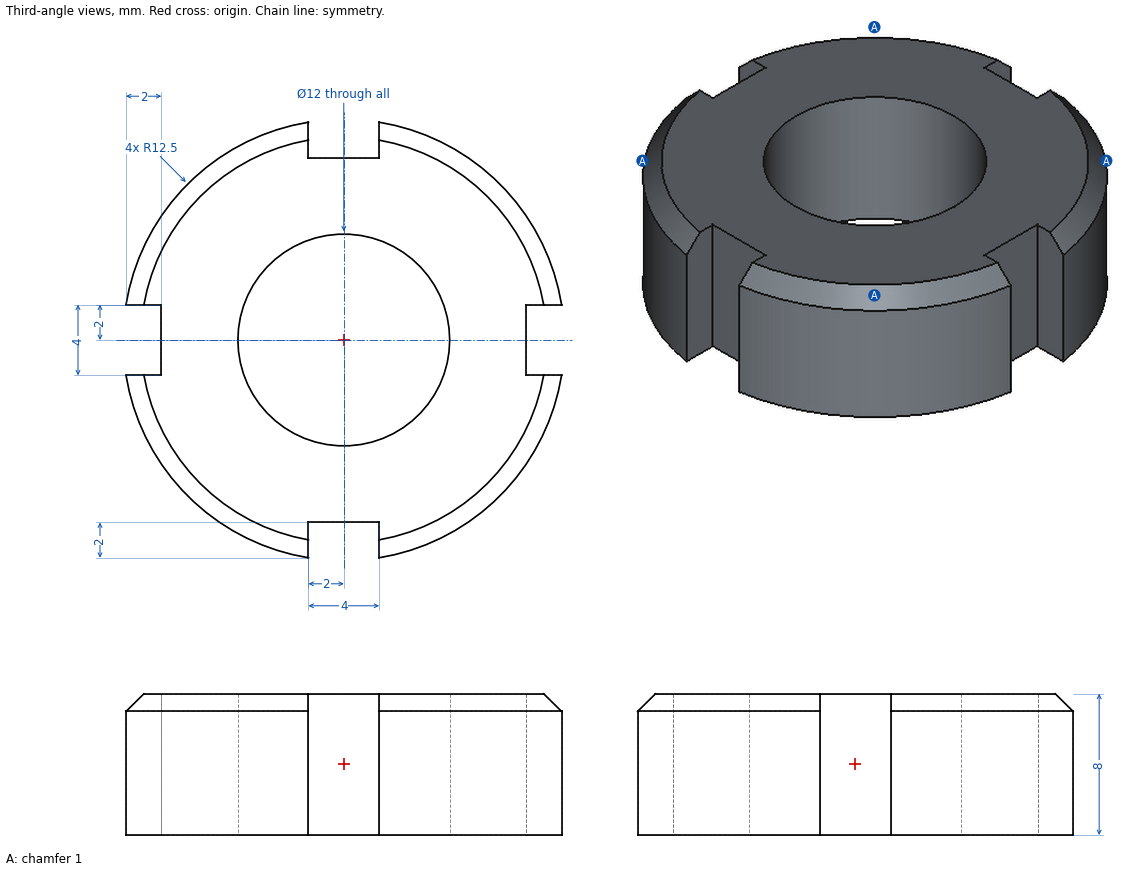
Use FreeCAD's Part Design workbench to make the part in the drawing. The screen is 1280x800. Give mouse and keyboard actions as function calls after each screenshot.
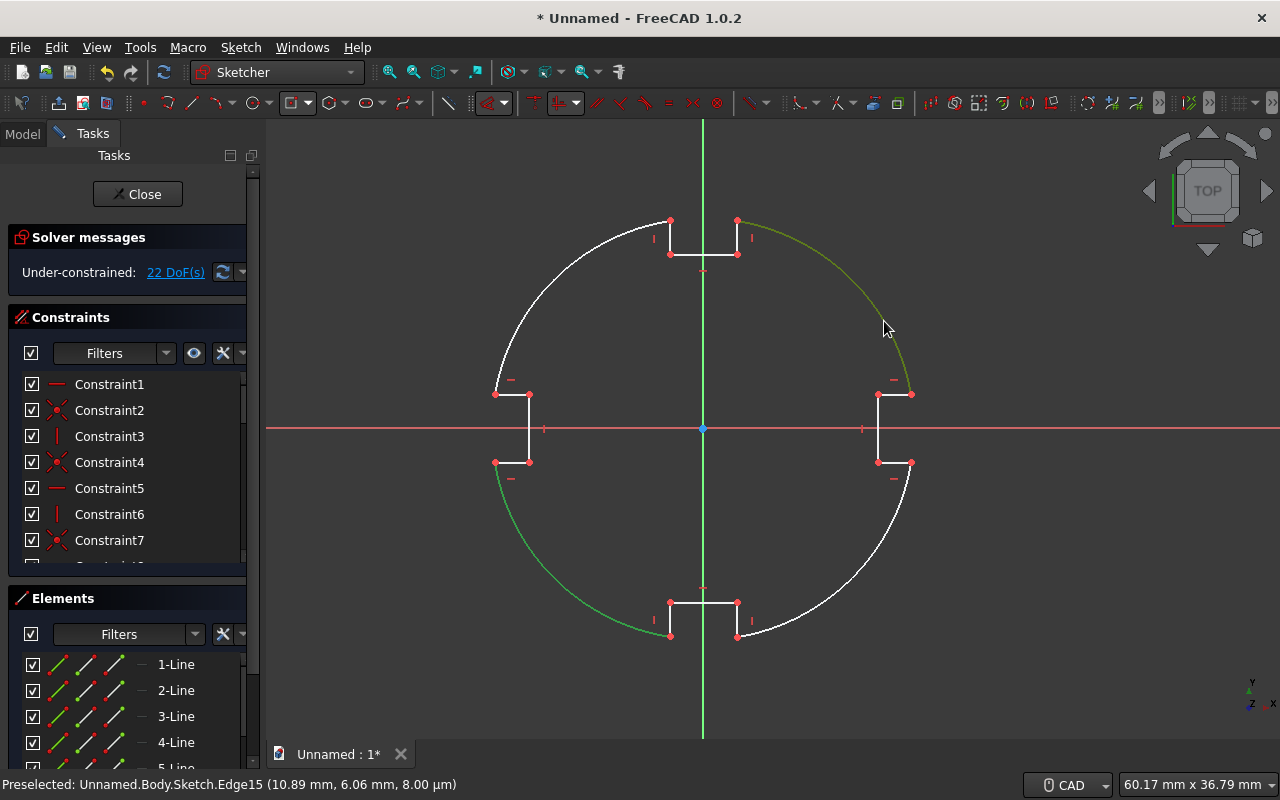
key(c)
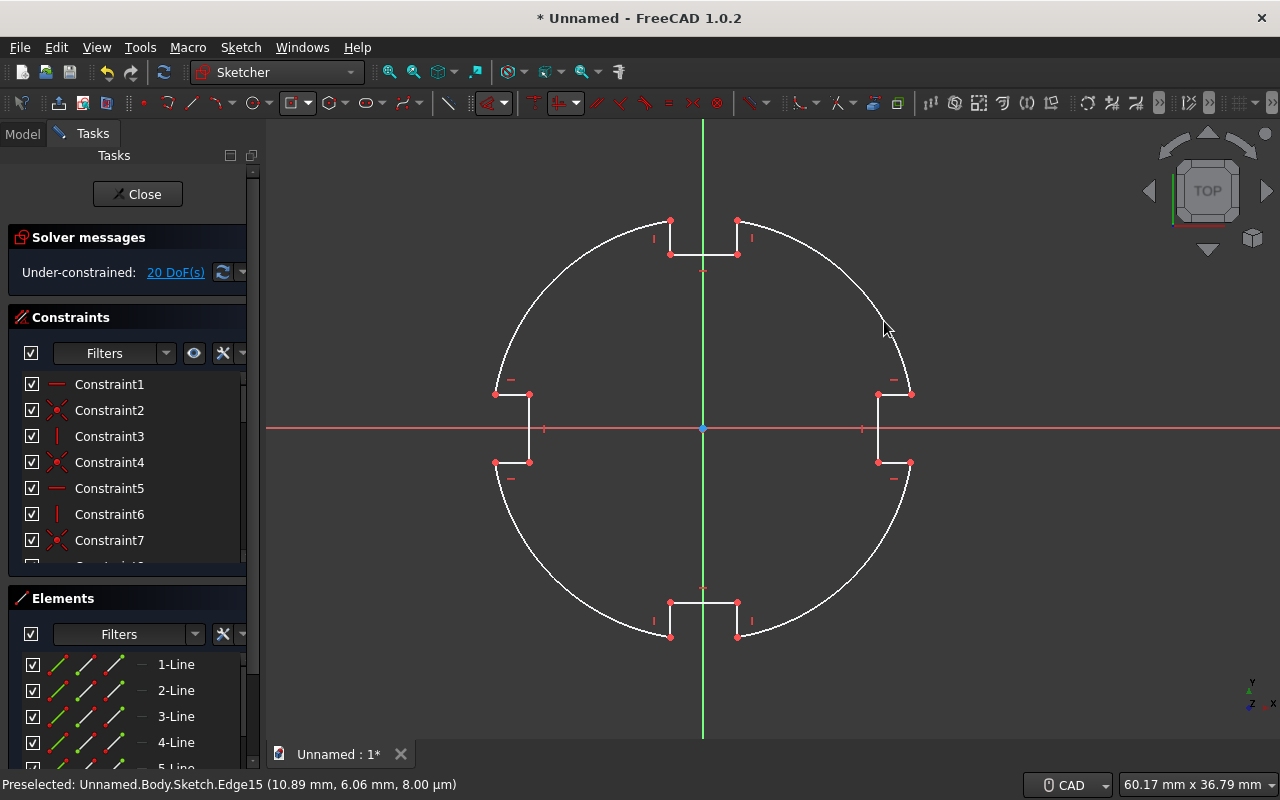
click(522, 537)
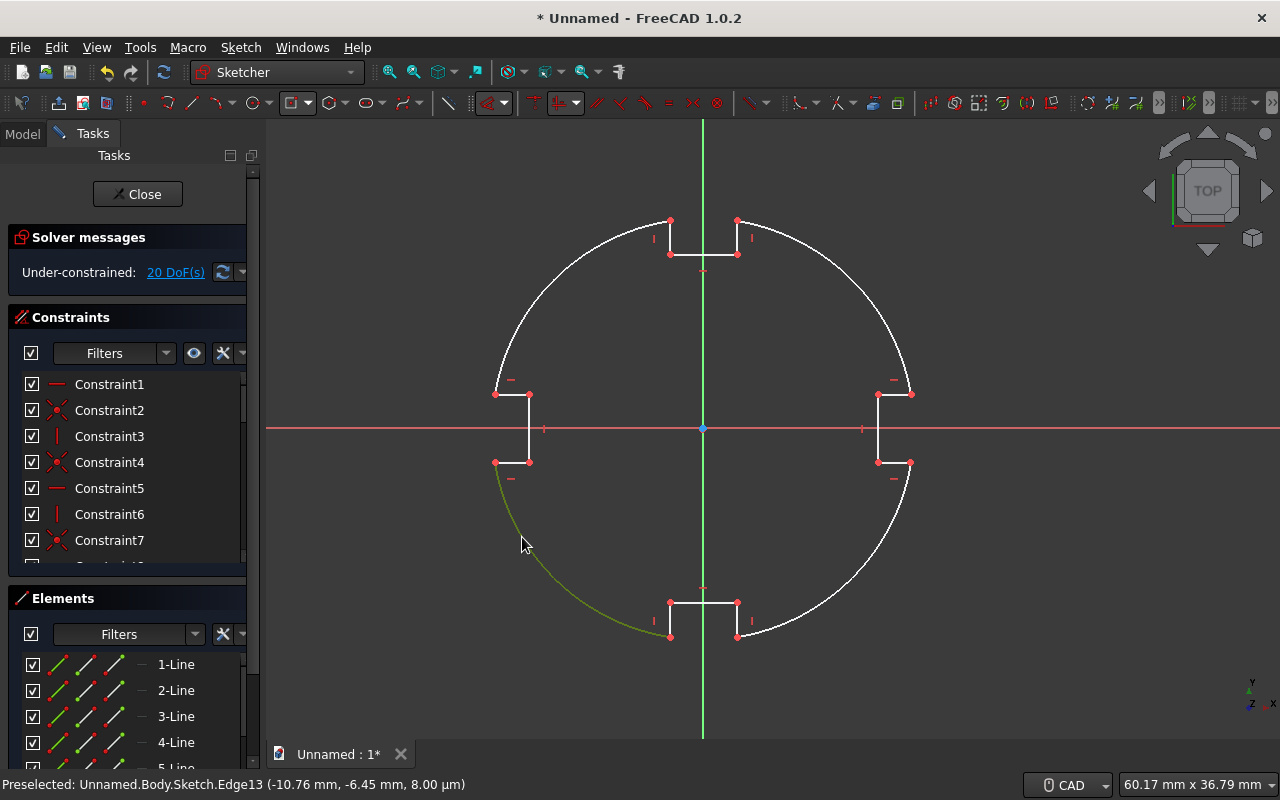
click(596, 248)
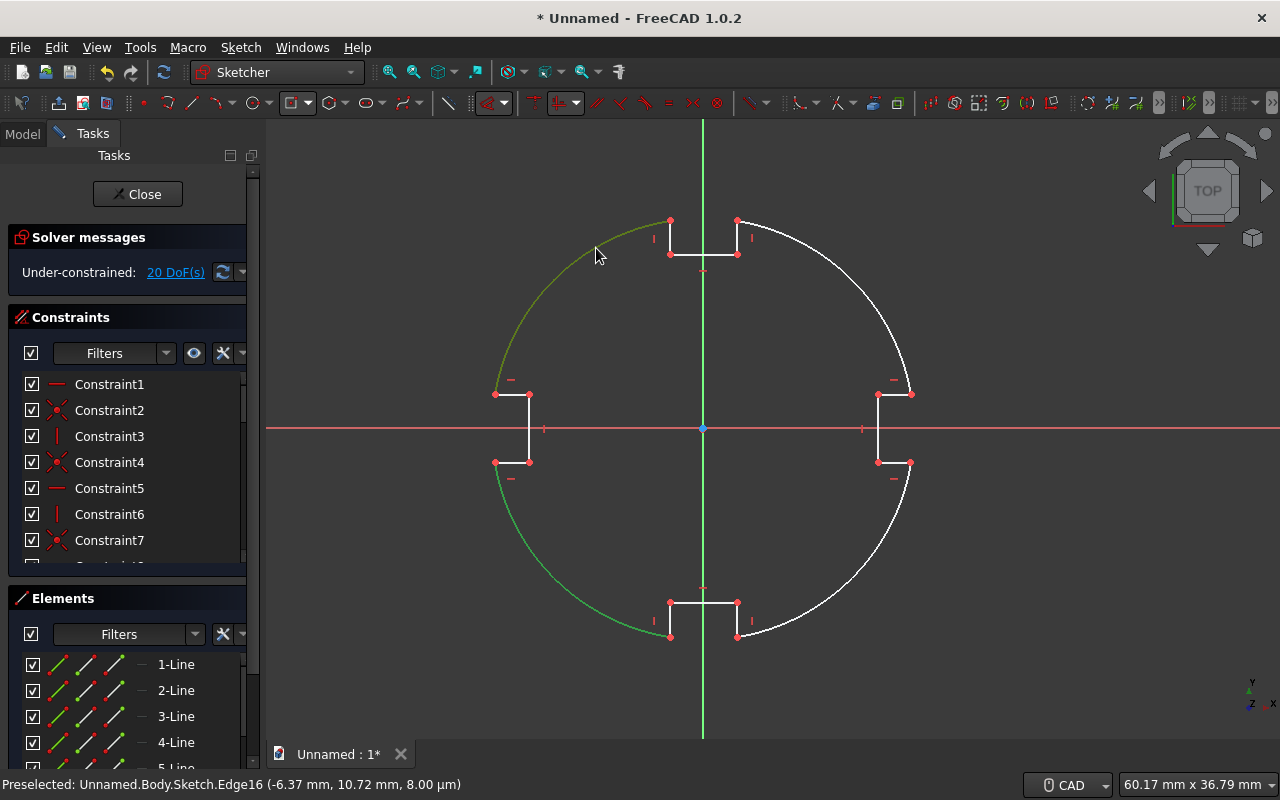
key(c)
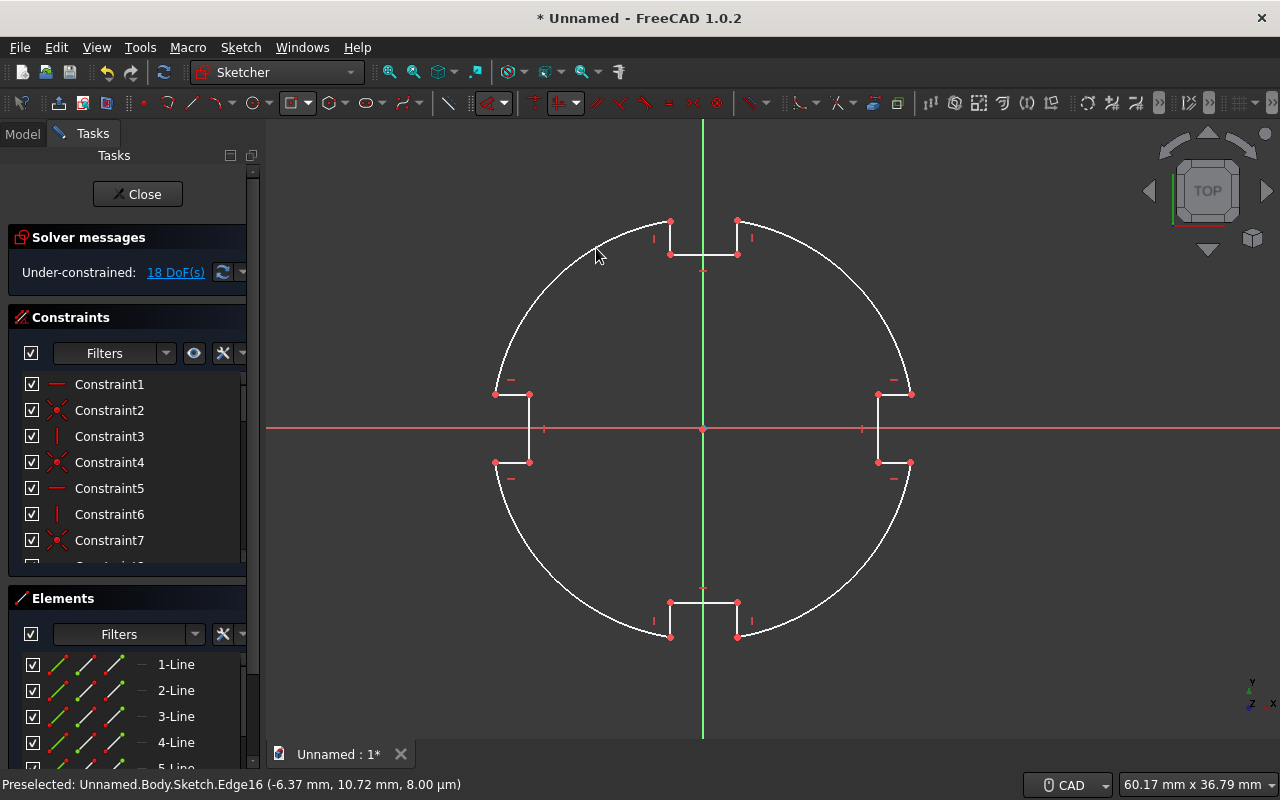
drag(693, 418, 713, 439)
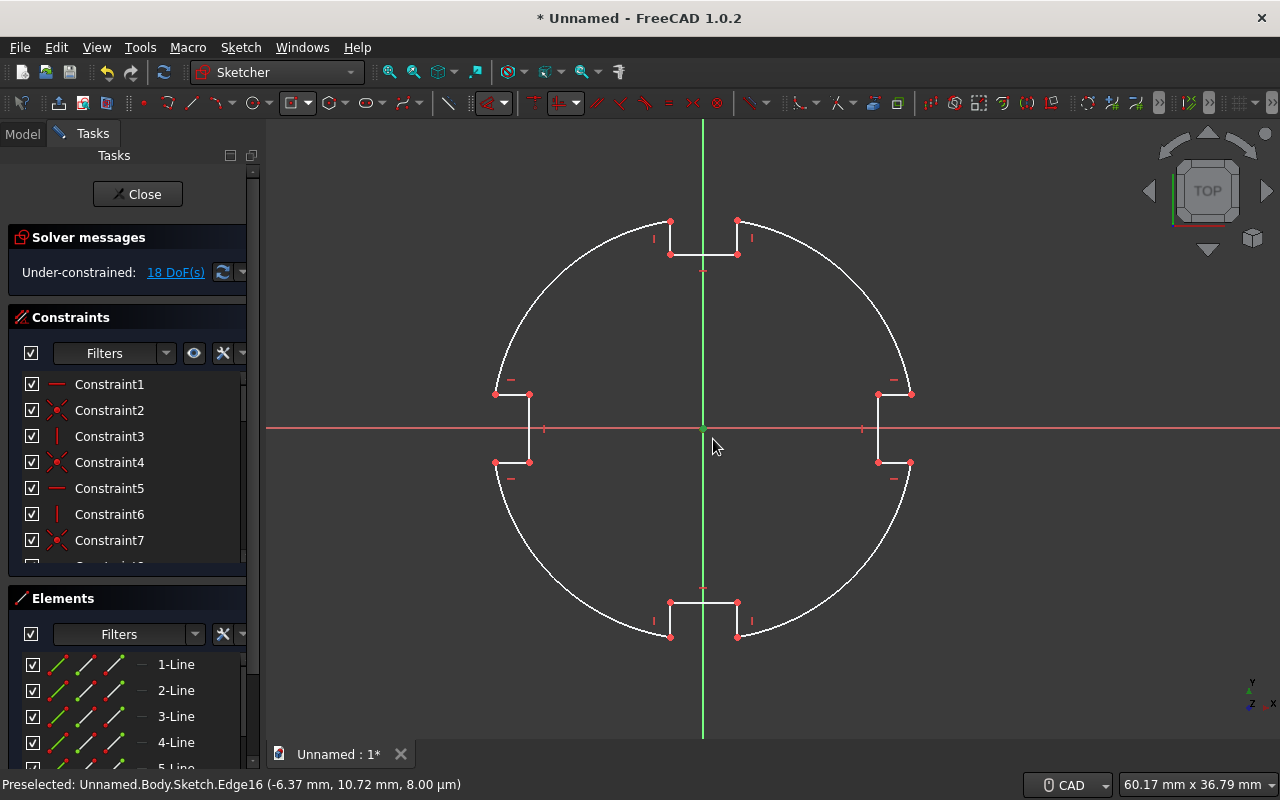
key(c)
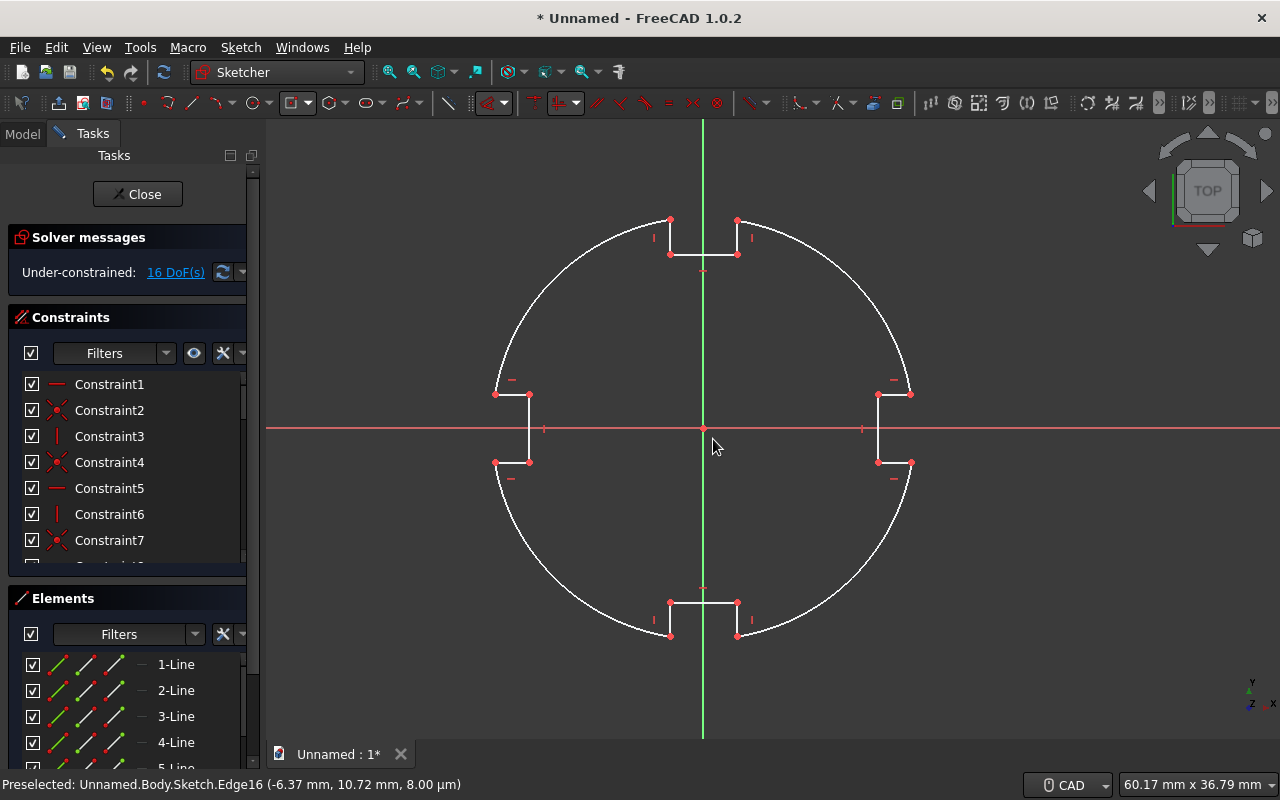
click(522, 537)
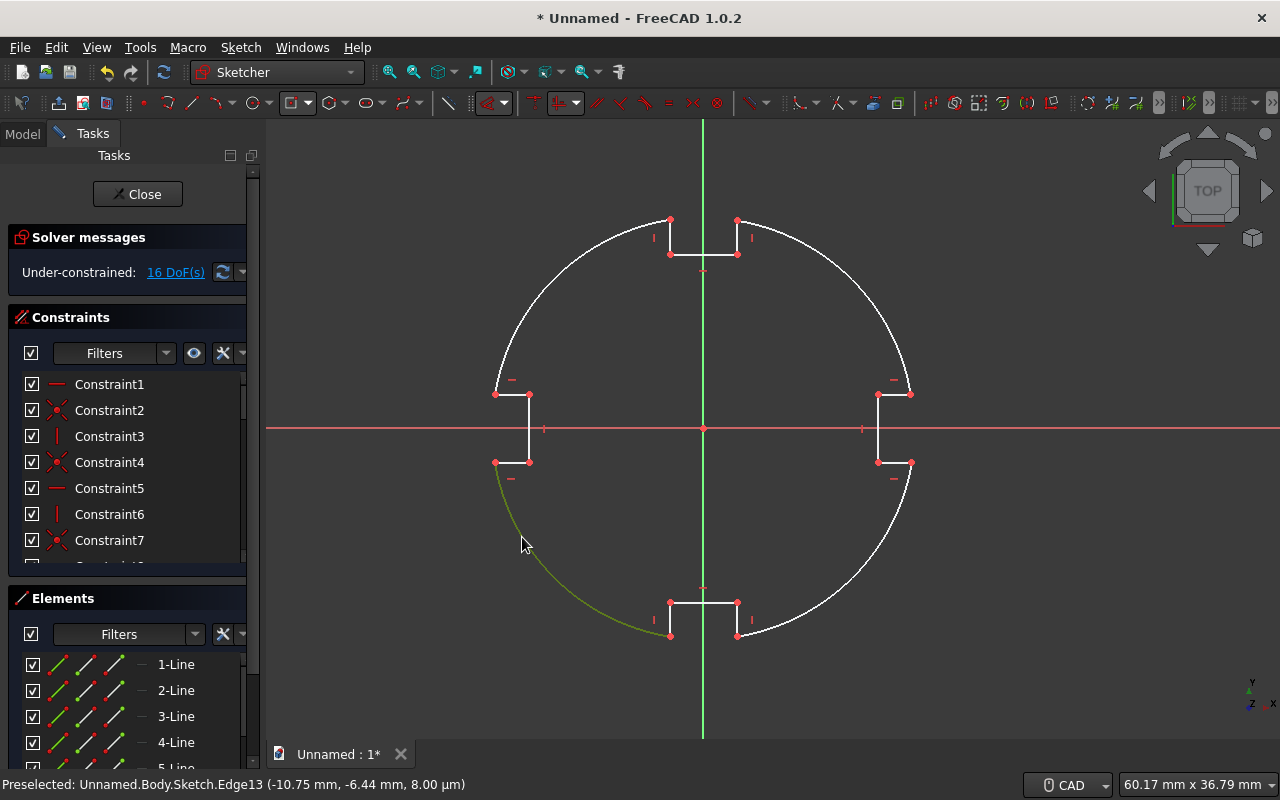
click(811, 610)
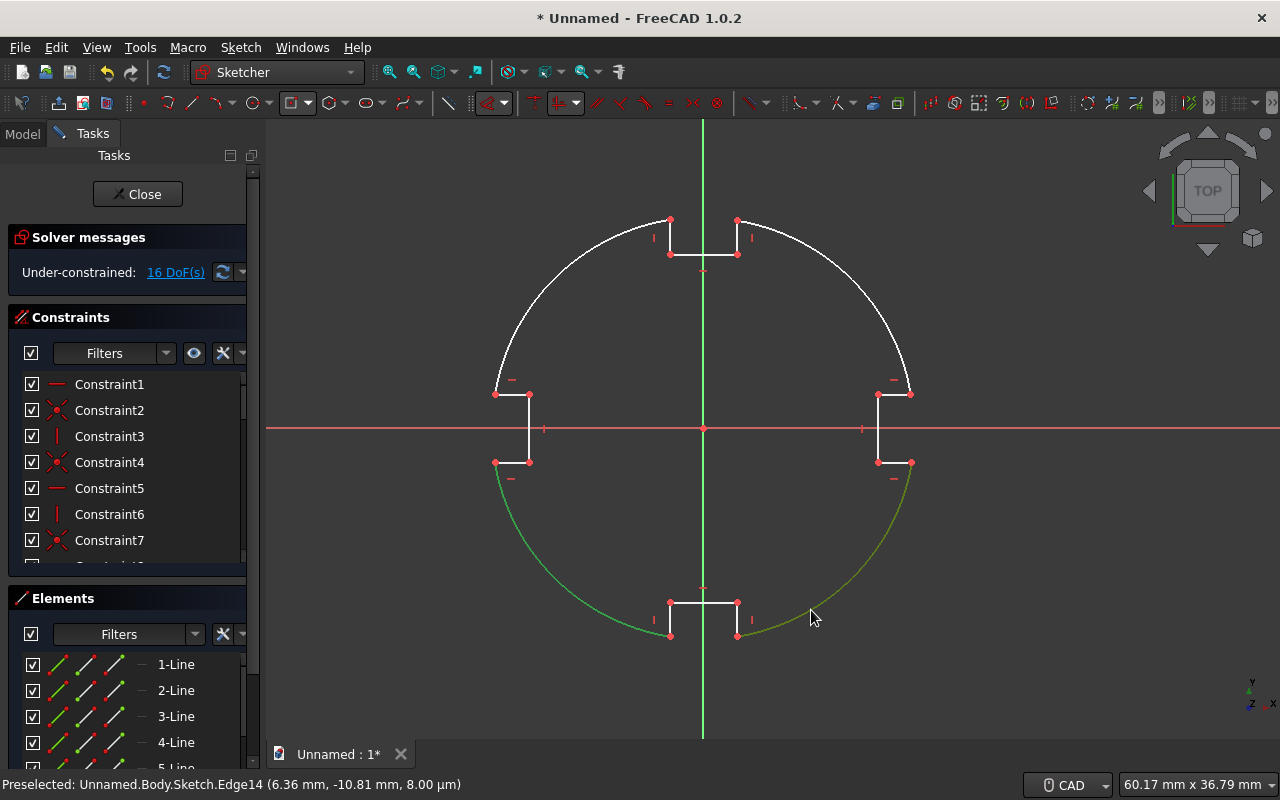
click(884, 321)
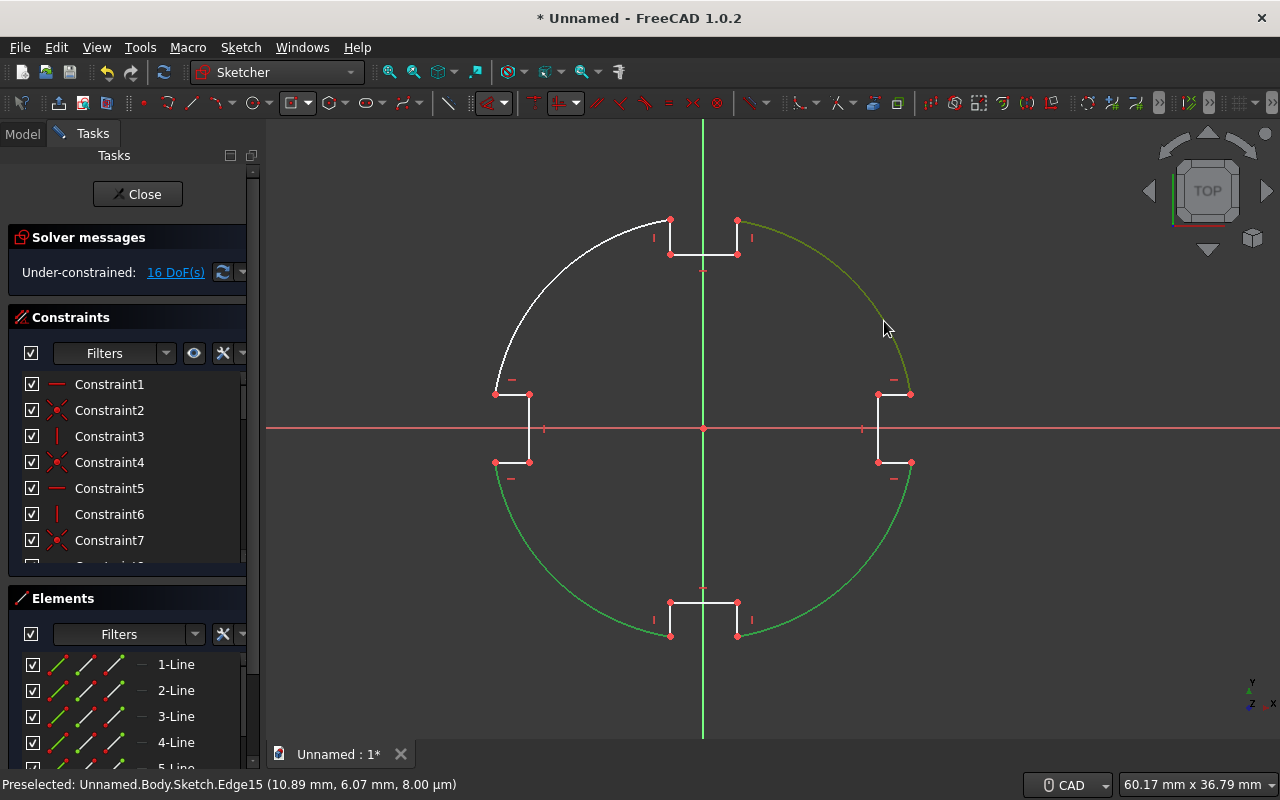
click(596, 247)